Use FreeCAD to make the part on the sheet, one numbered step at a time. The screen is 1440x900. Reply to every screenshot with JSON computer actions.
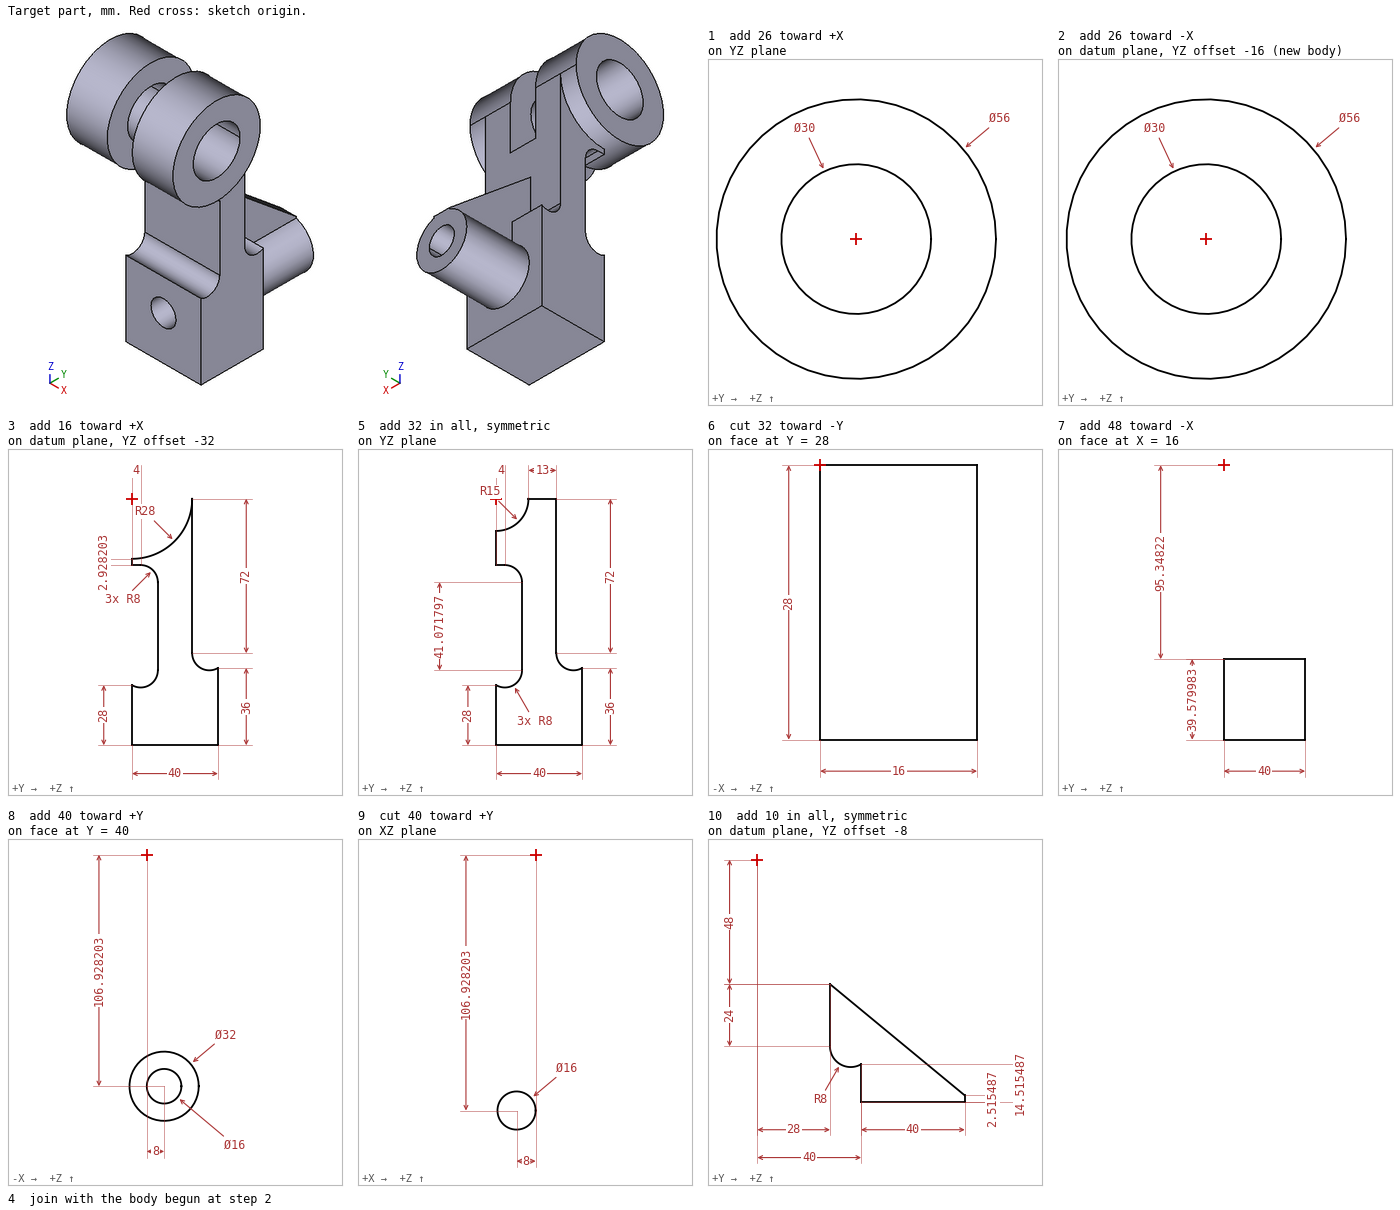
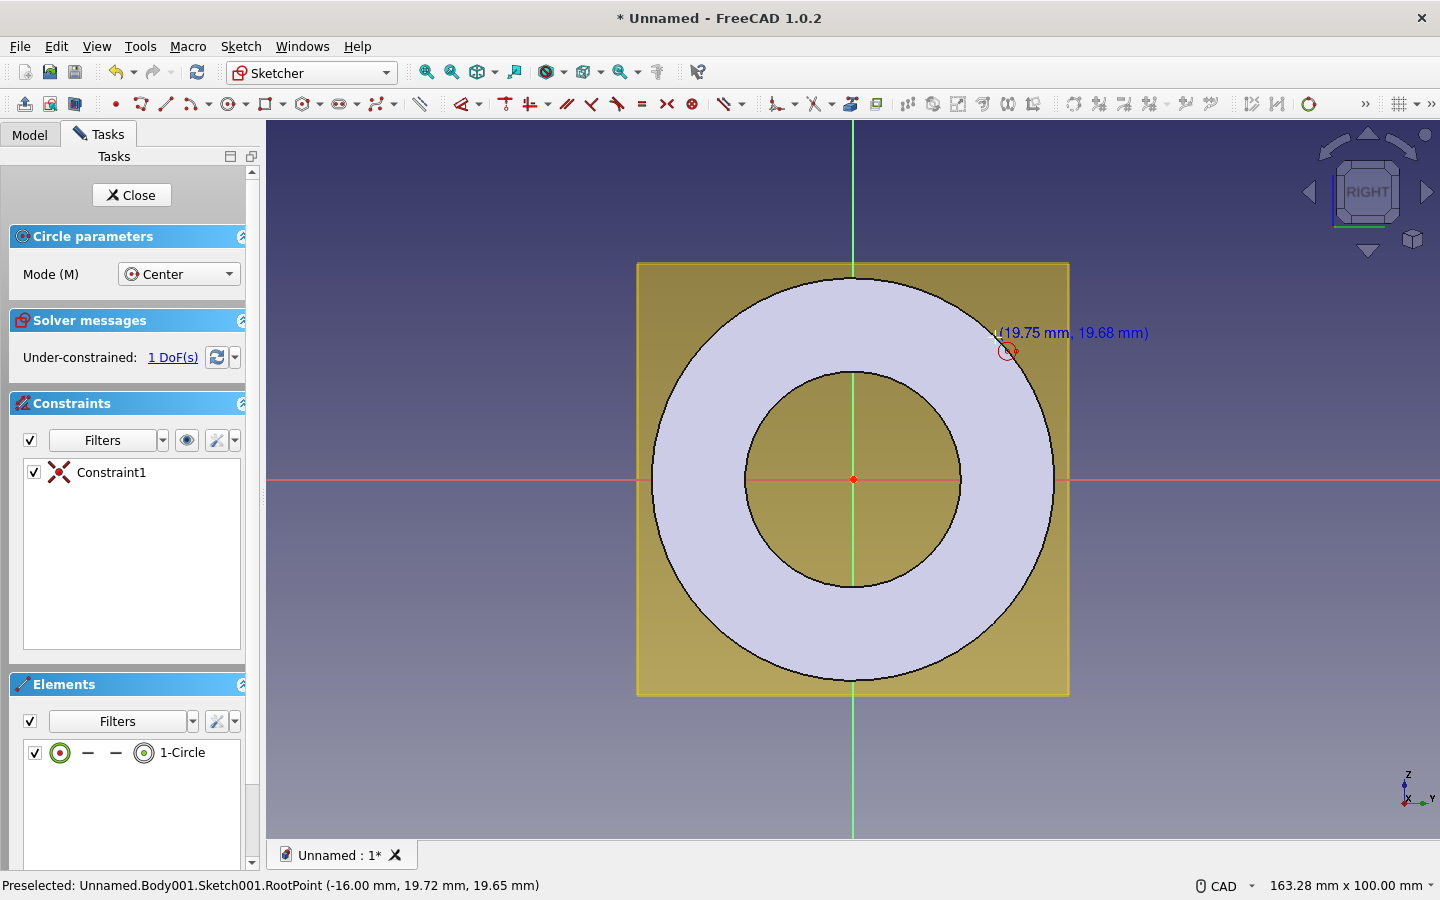
{"action": "left_click", "coordinate": [853, 480]}
{"action": "left_click", "coordinate": [929, 403]}
{"action": "key", "text": "Escape"}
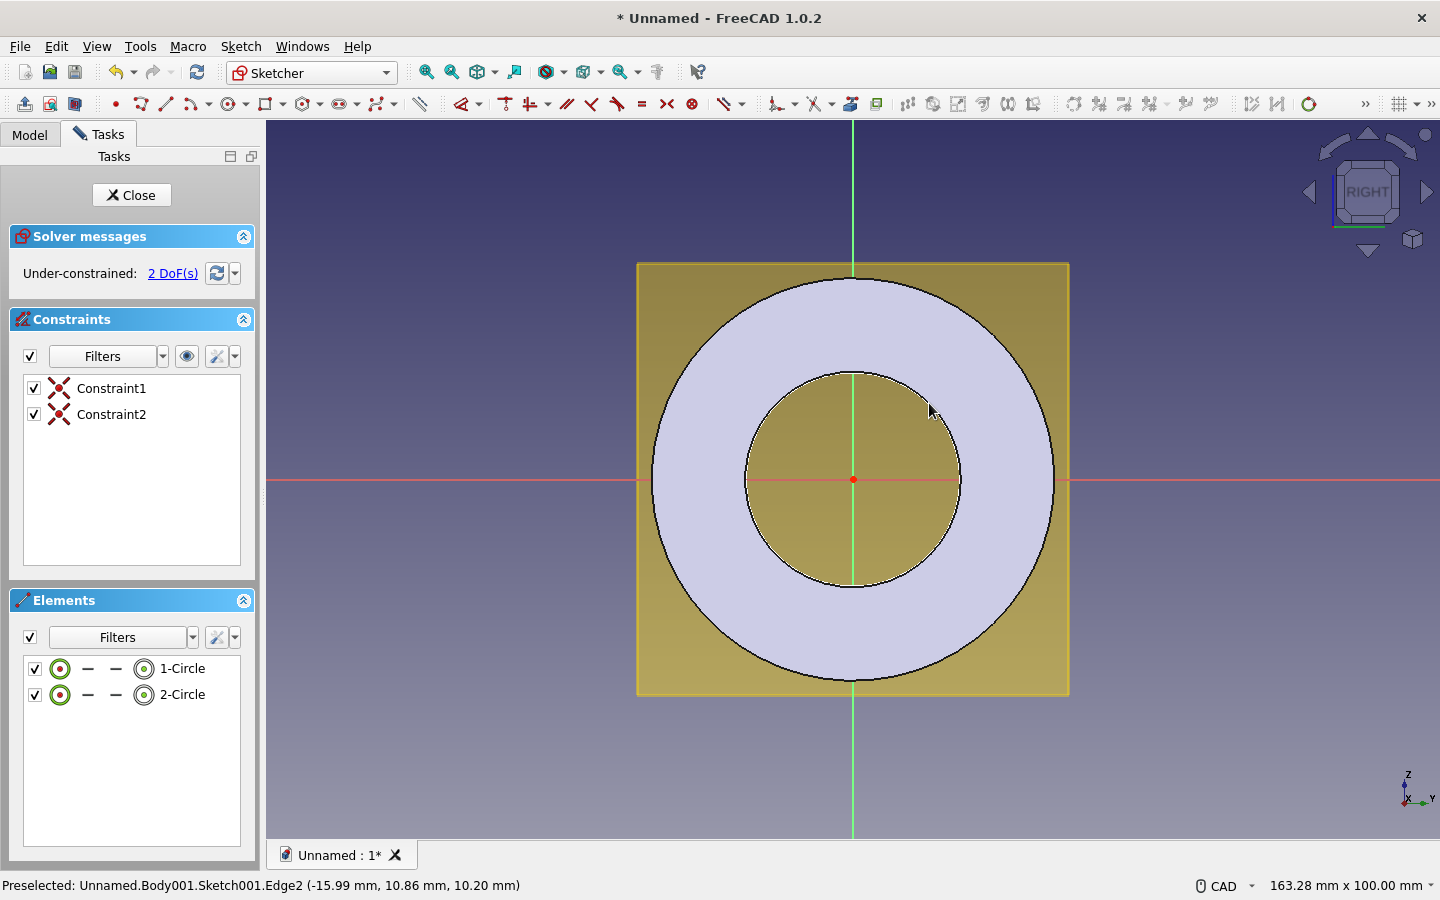
{"action": "key", "text": "d"}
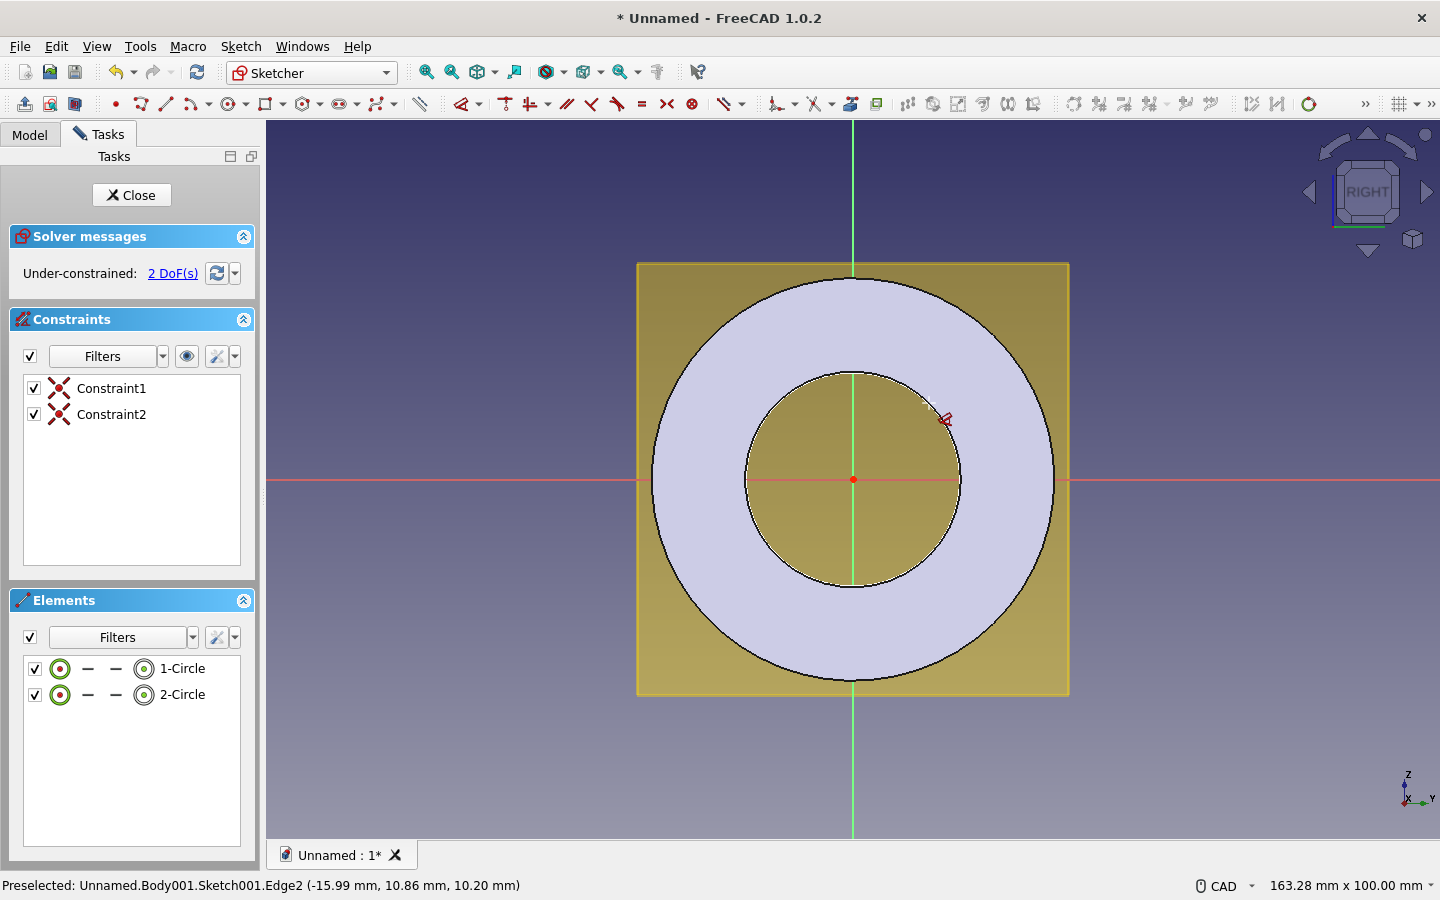
{"action": "left_click", "coordinate": [994, 337]}
{"action": "left_click", "coordinate": [1017, 314]}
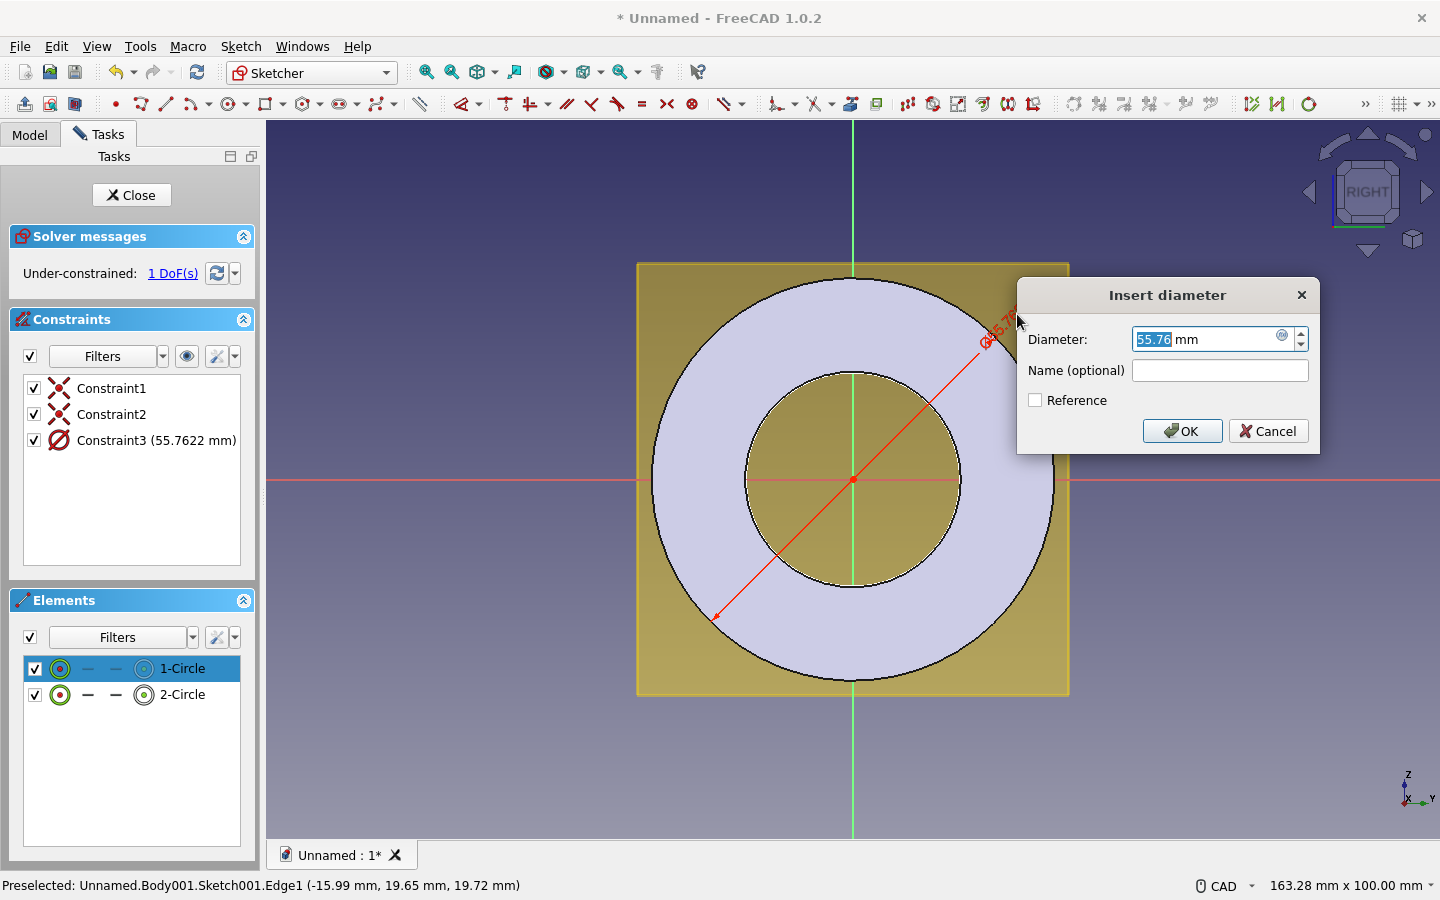
{"action": "type", "text": "56"}
{"action": "key", "text": "Return"}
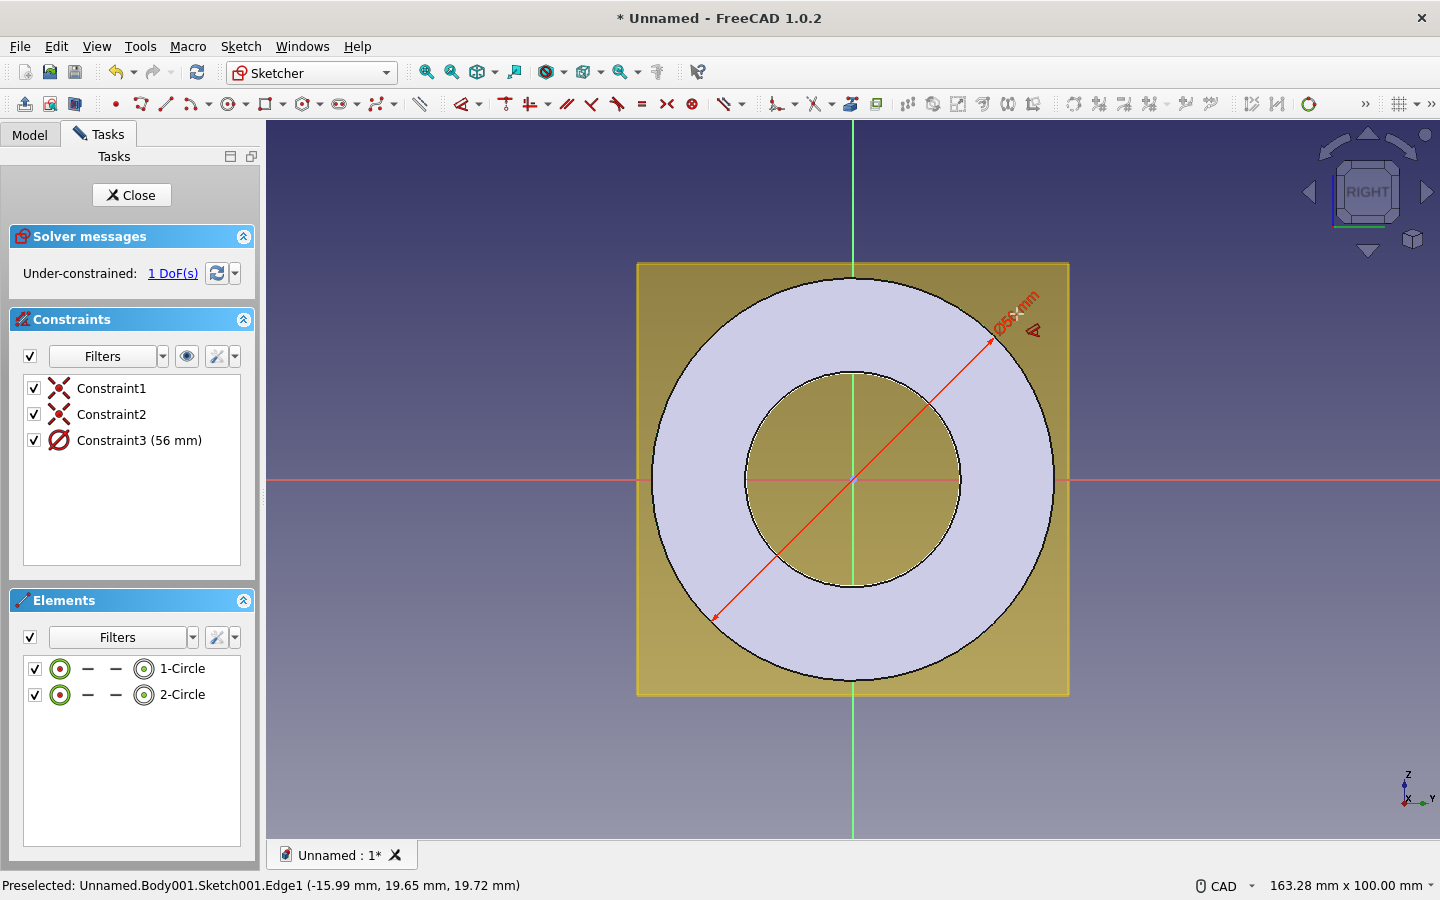
{"action": "left_click", "coordinate": [929, 404]}
{"action": "left_click", "coordinate": [952, 381]}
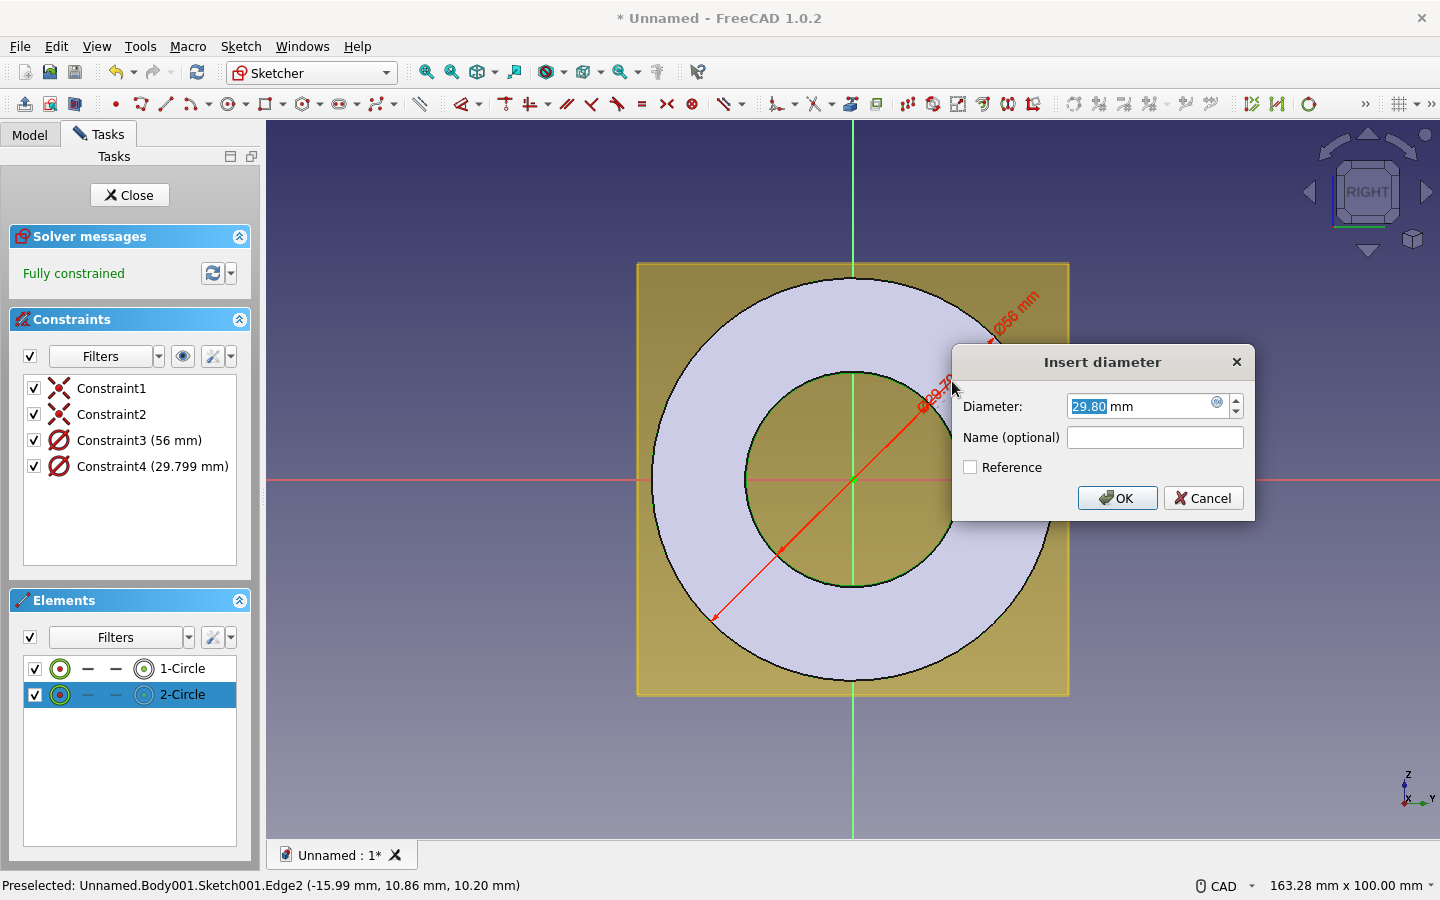
{"action": "type", "text": "30"}
{"action": "key", "text": "Return"}
{"action": "key", "text": "Escape"}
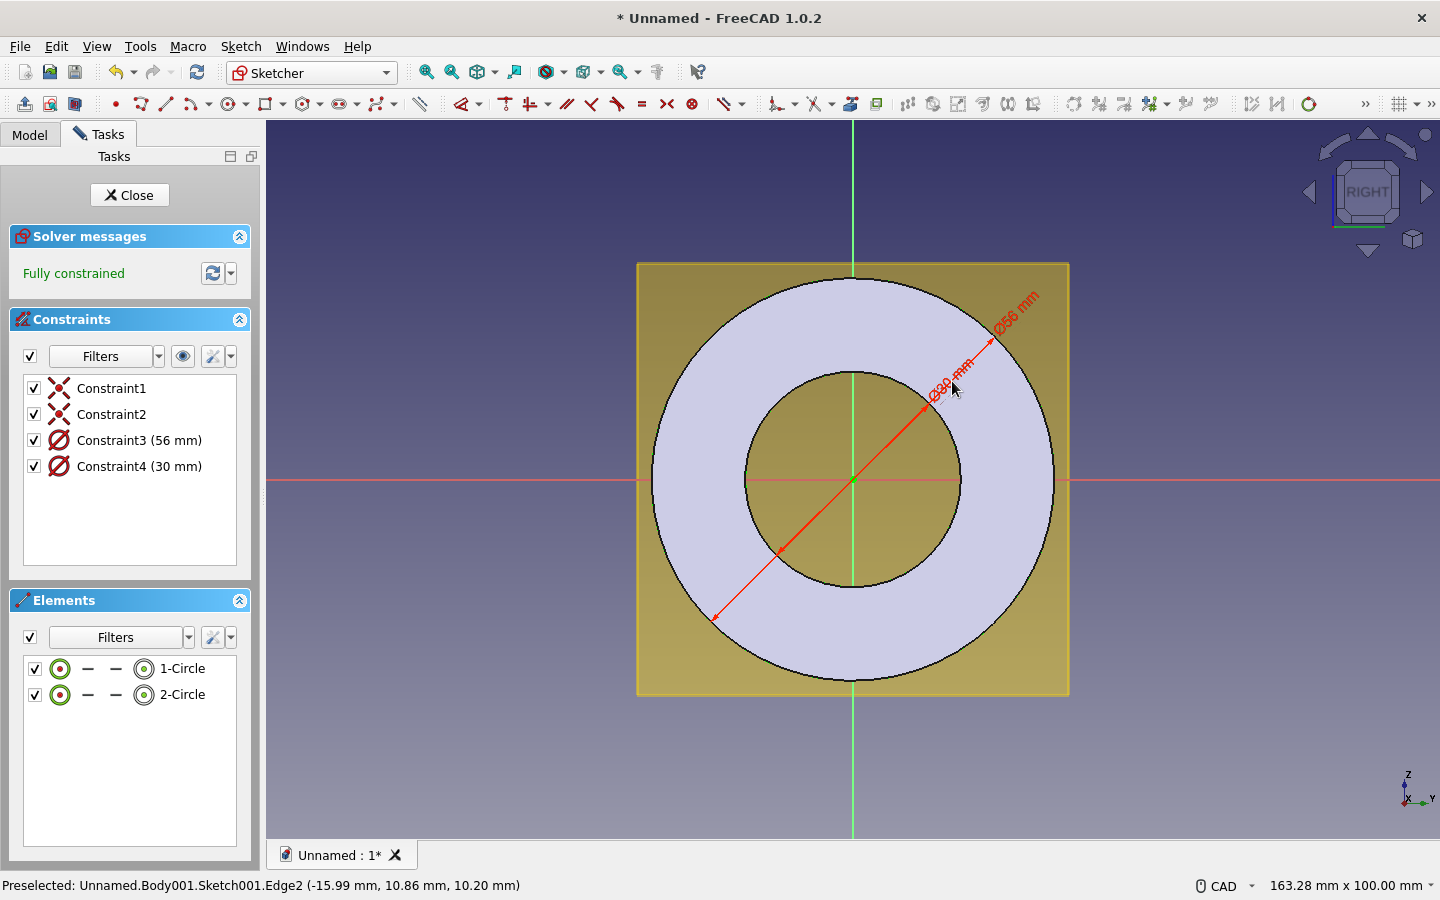
{"action": "left_click", "coordinate": [130, 195]}